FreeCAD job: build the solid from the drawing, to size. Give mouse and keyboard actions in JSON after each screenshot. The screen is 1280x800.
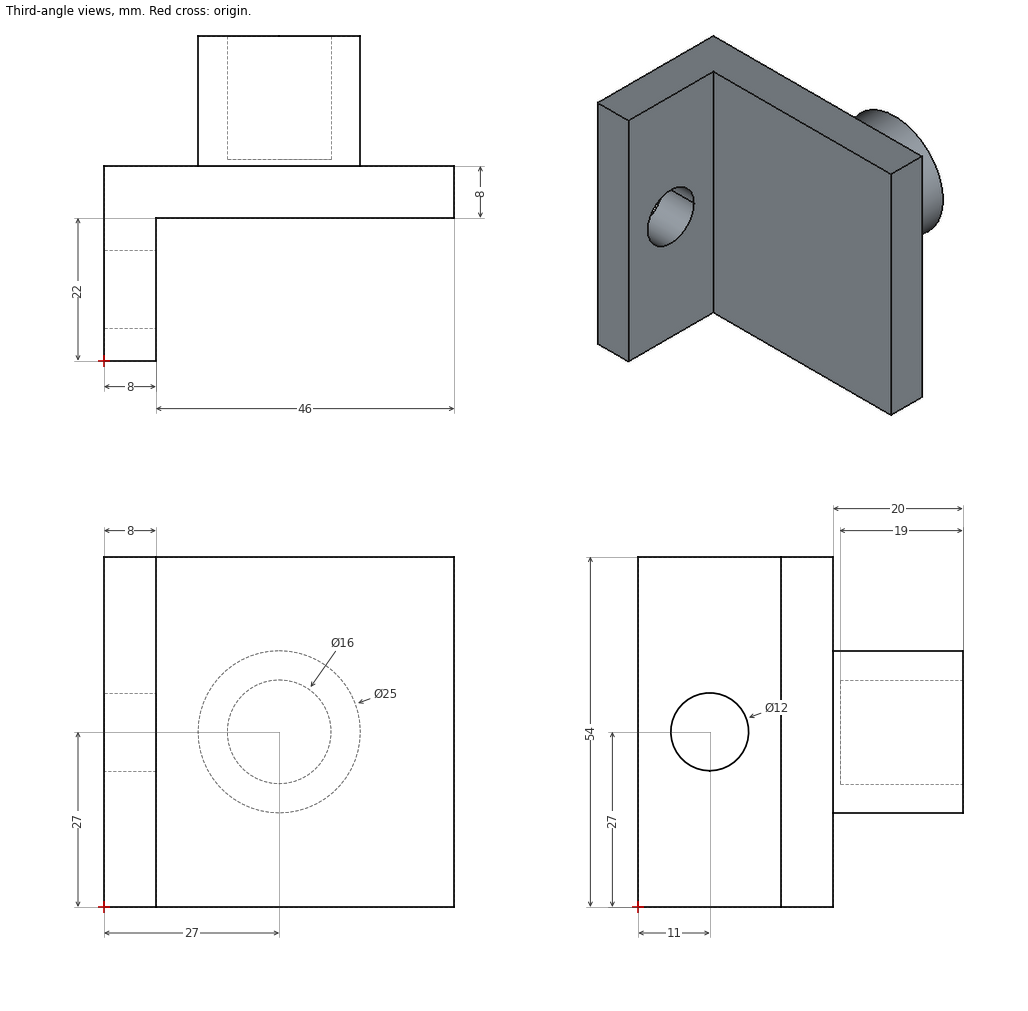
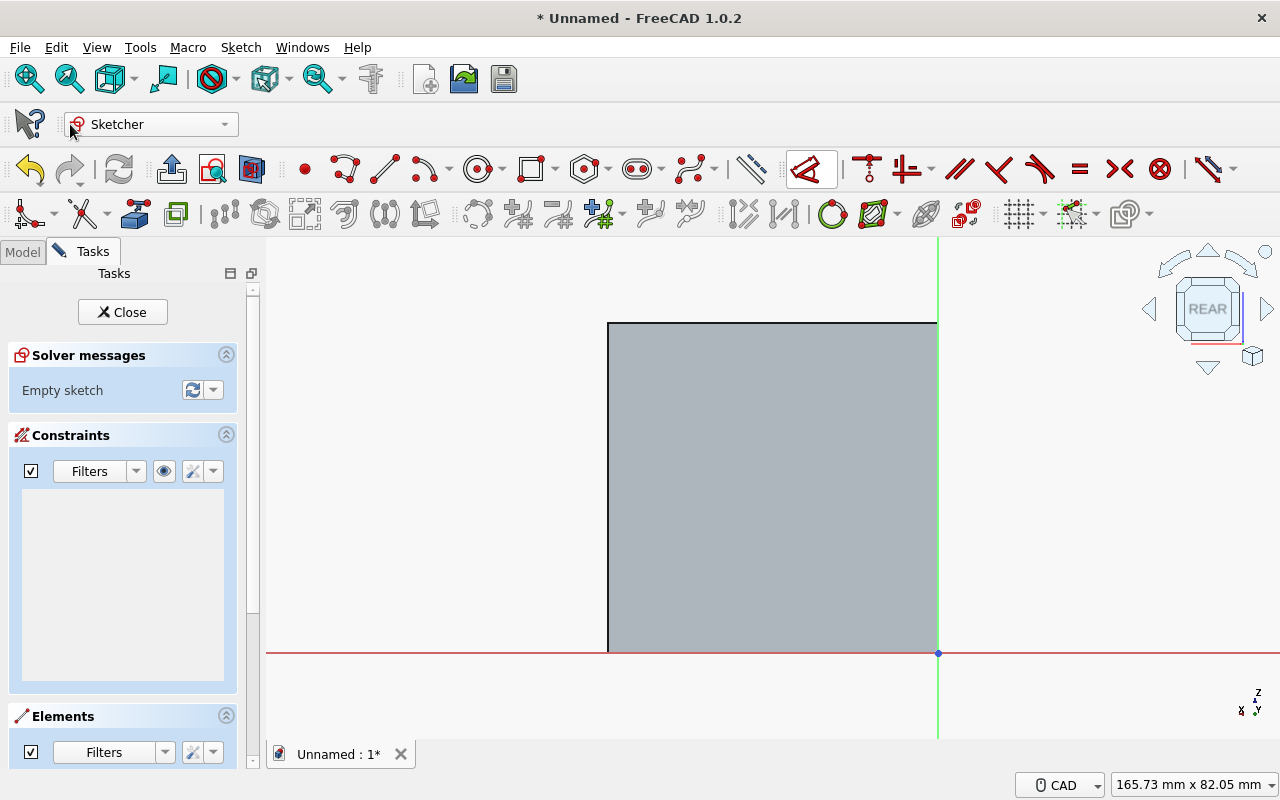
{"action": "key", "text": "g c"}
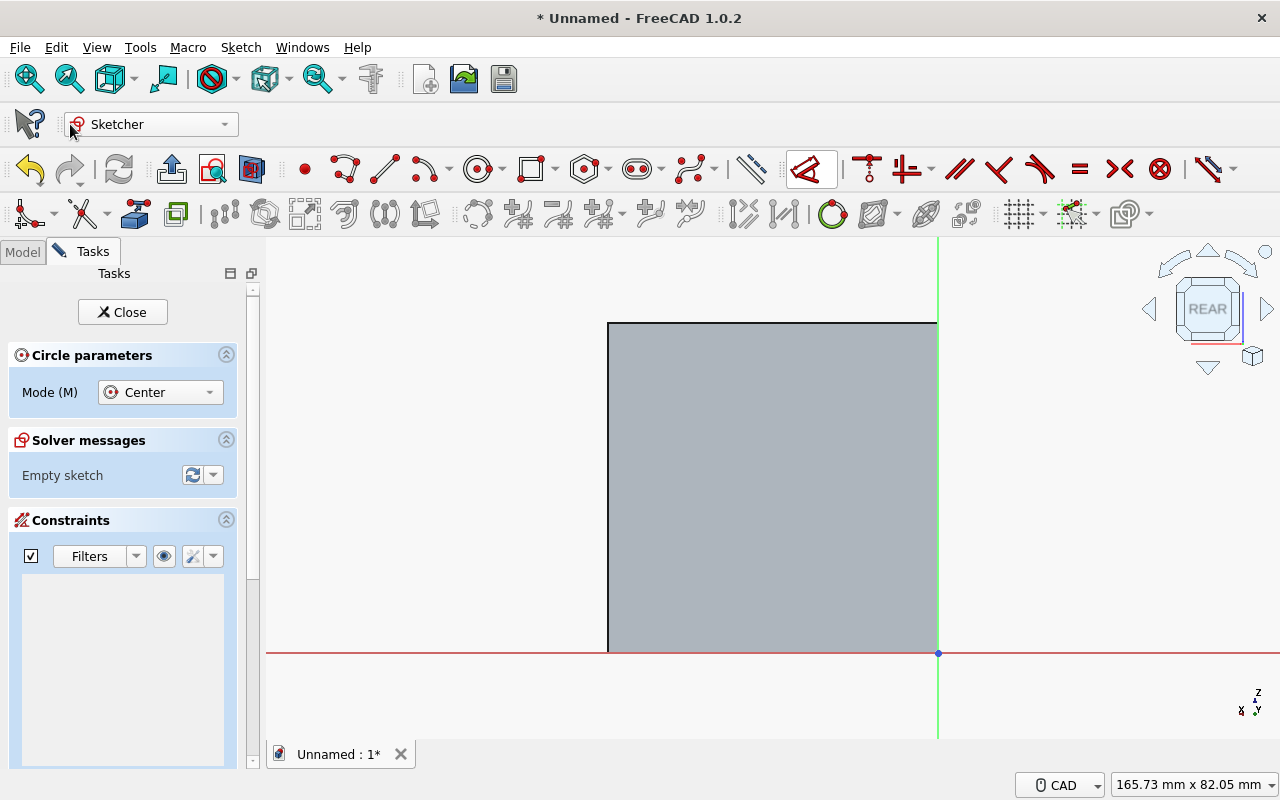
{"action": "left_click", "coordinate": [773, 488]}
{"action": "mouse_move", "coordinate": [827, 434]}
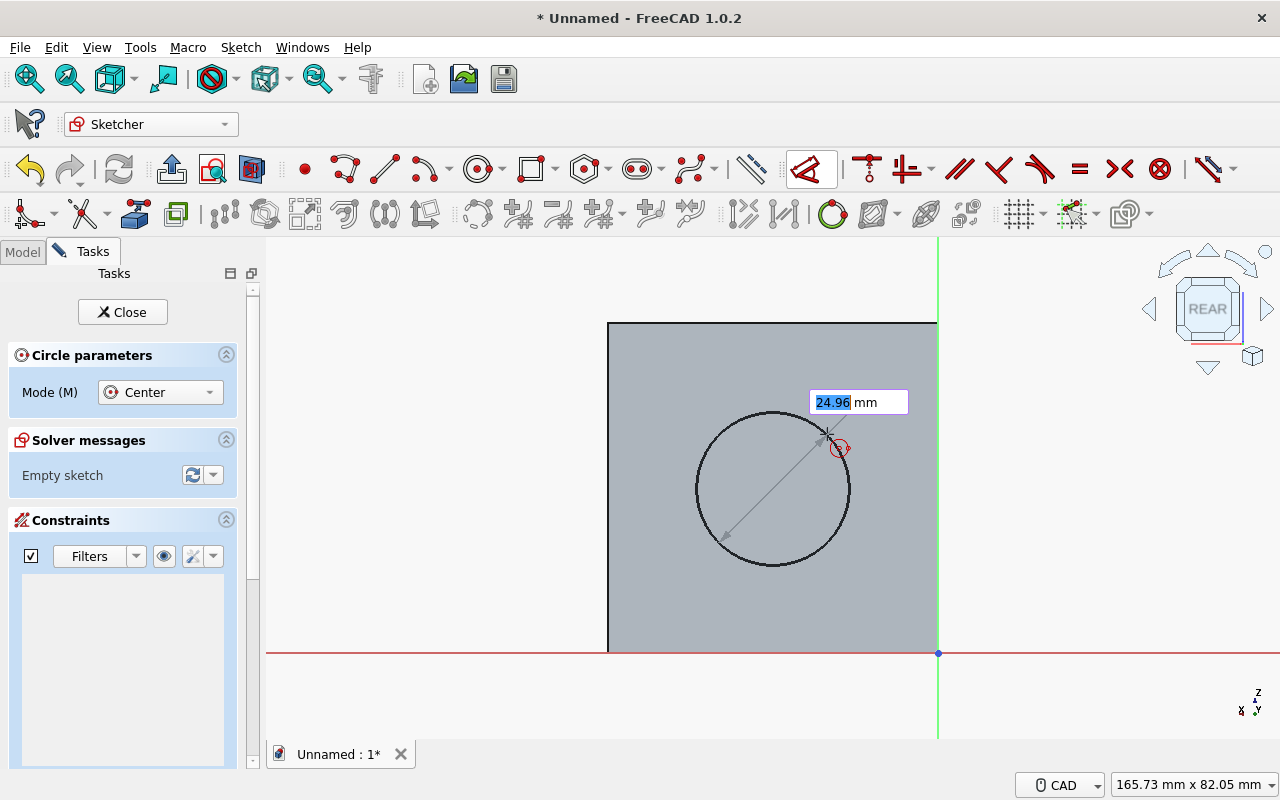
{"action": "type", "text": "25"}
{"action": "key", "text": "Return"}
{"action": "key", "text": "Escape"}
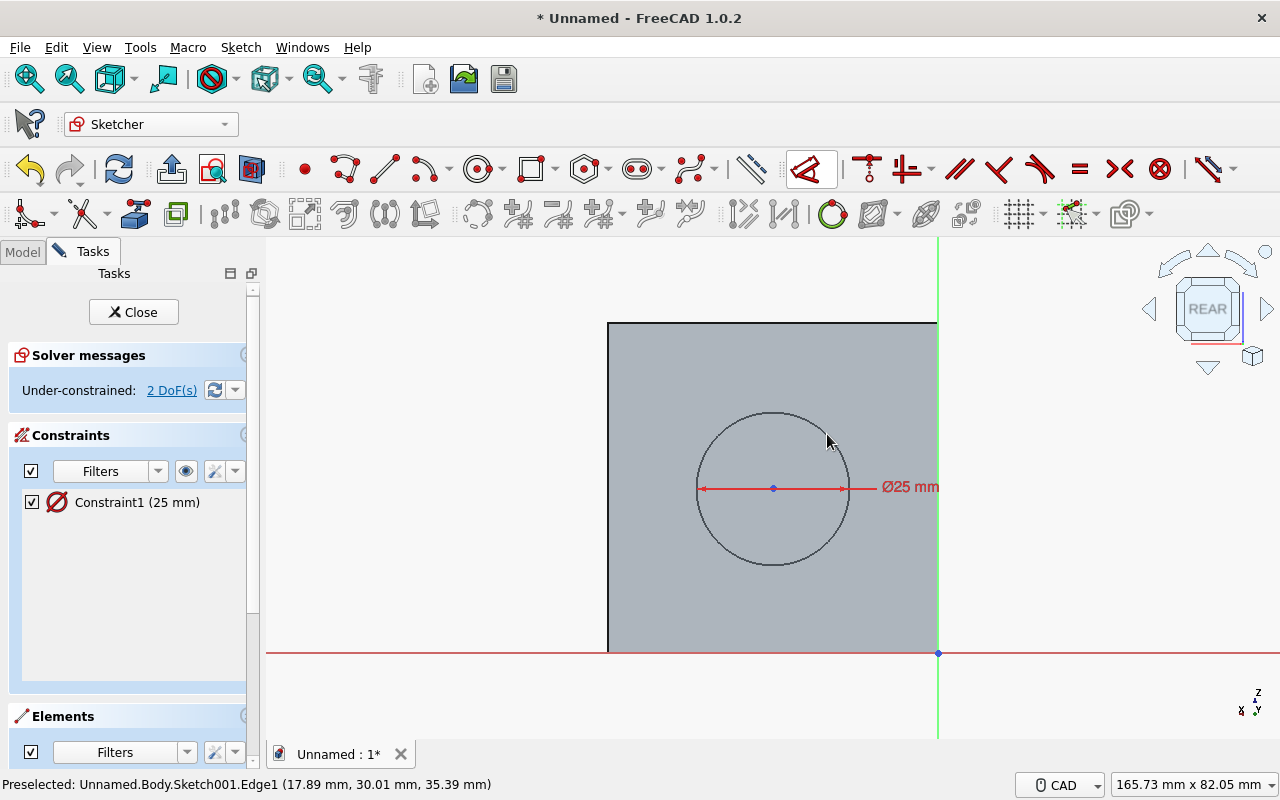
{"action": "left_click", "coordinate": [773, 489]}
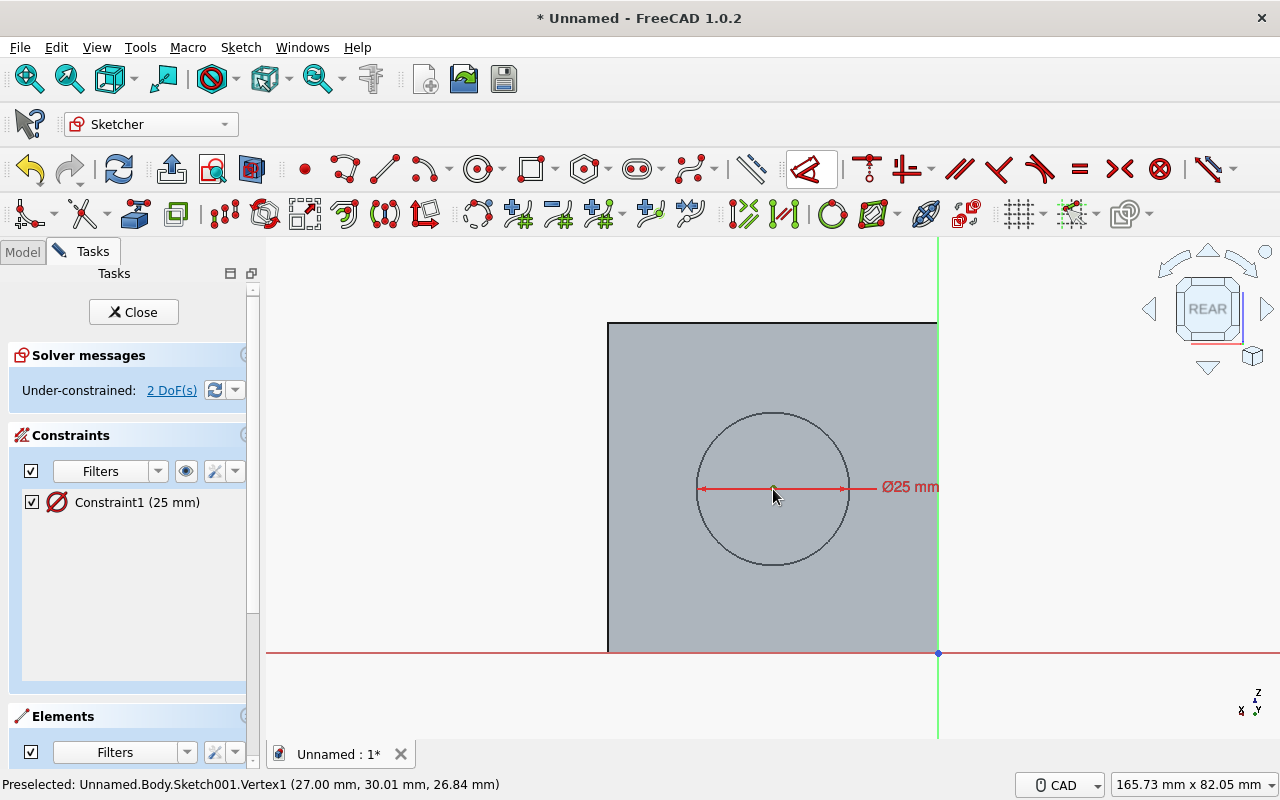
{"action": "key", "text": "l"}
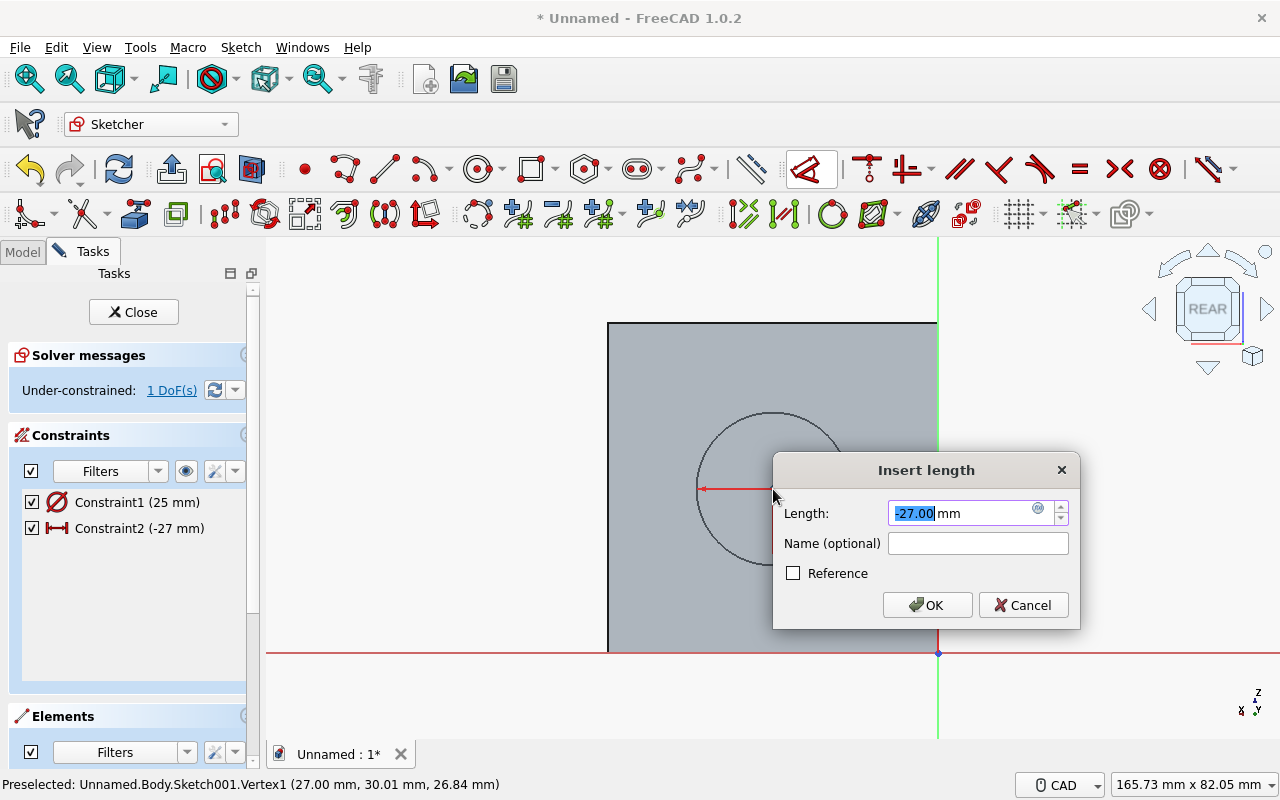
{"action": "type", "text": "-27"}
{"action": "key", "text": "Return"}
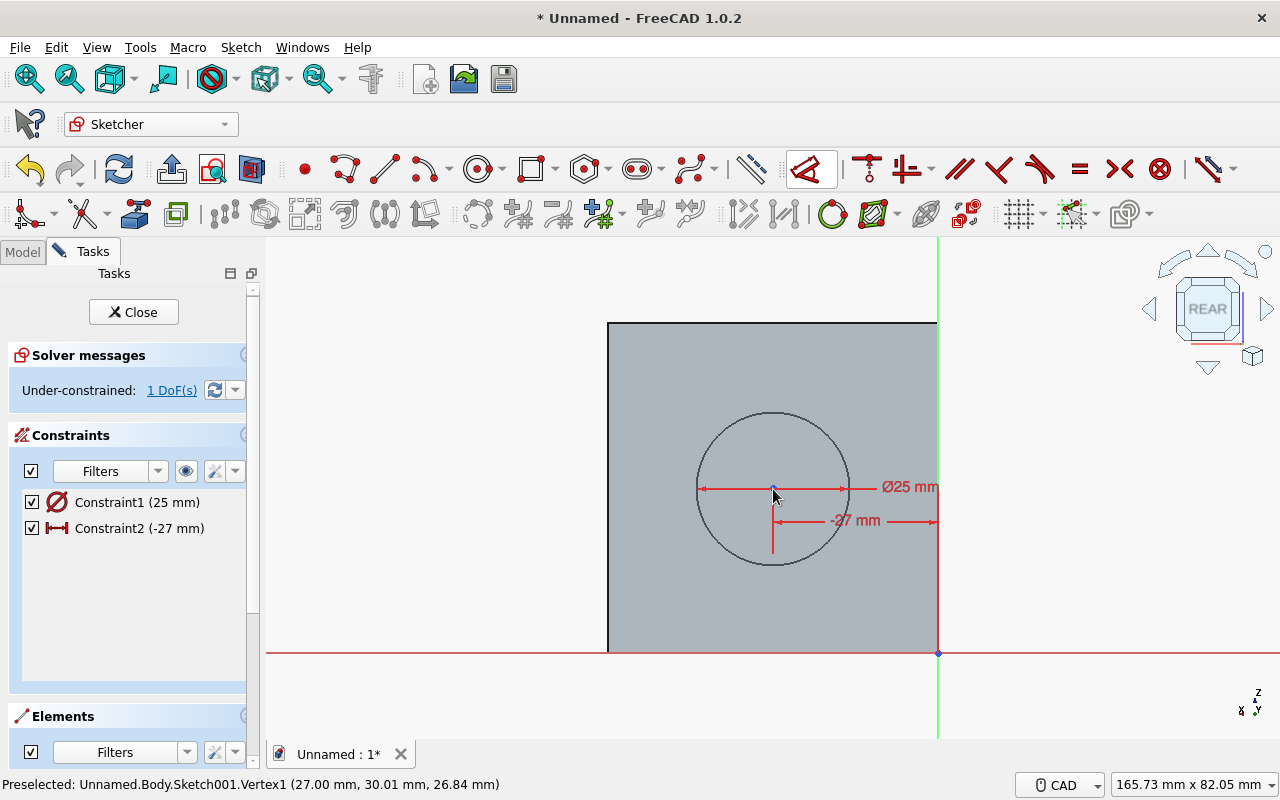
{"action": "left_click", "coordinate": [773, 489]}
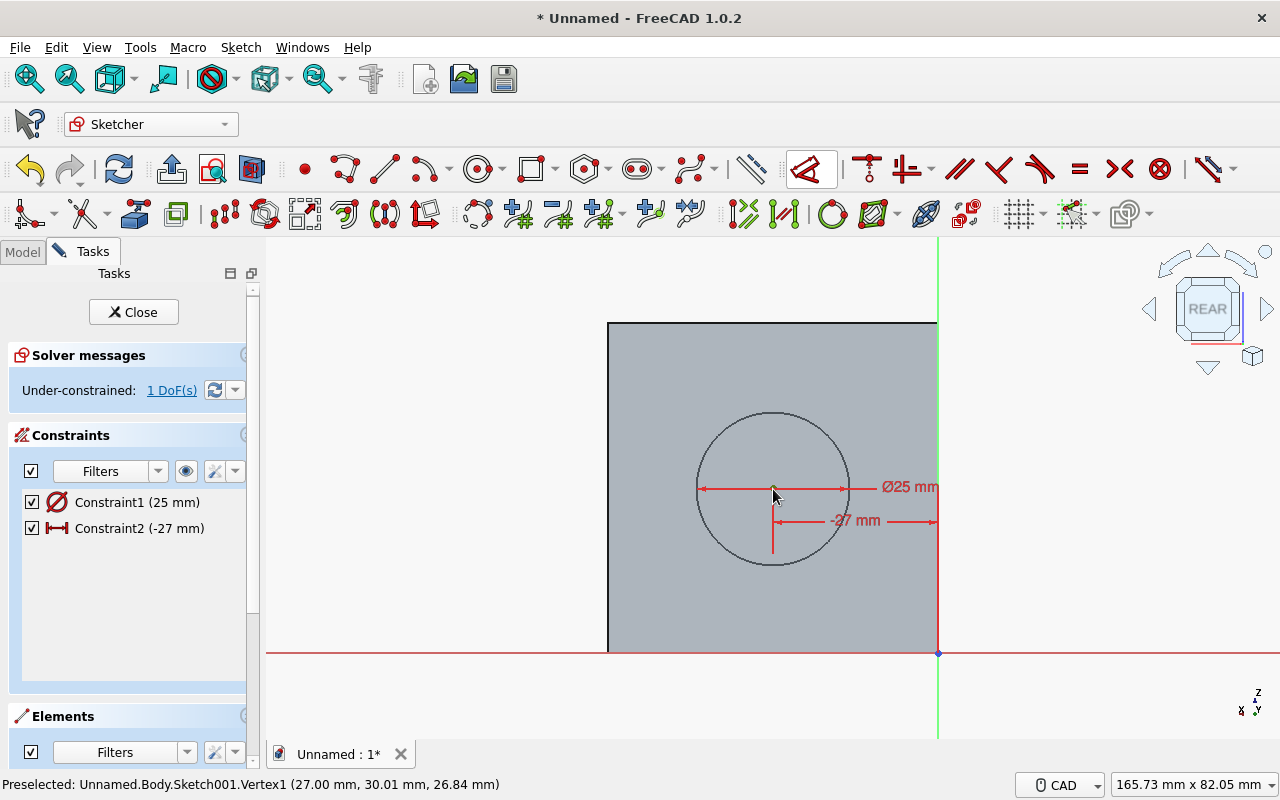
{"action": "key", "text": "i"}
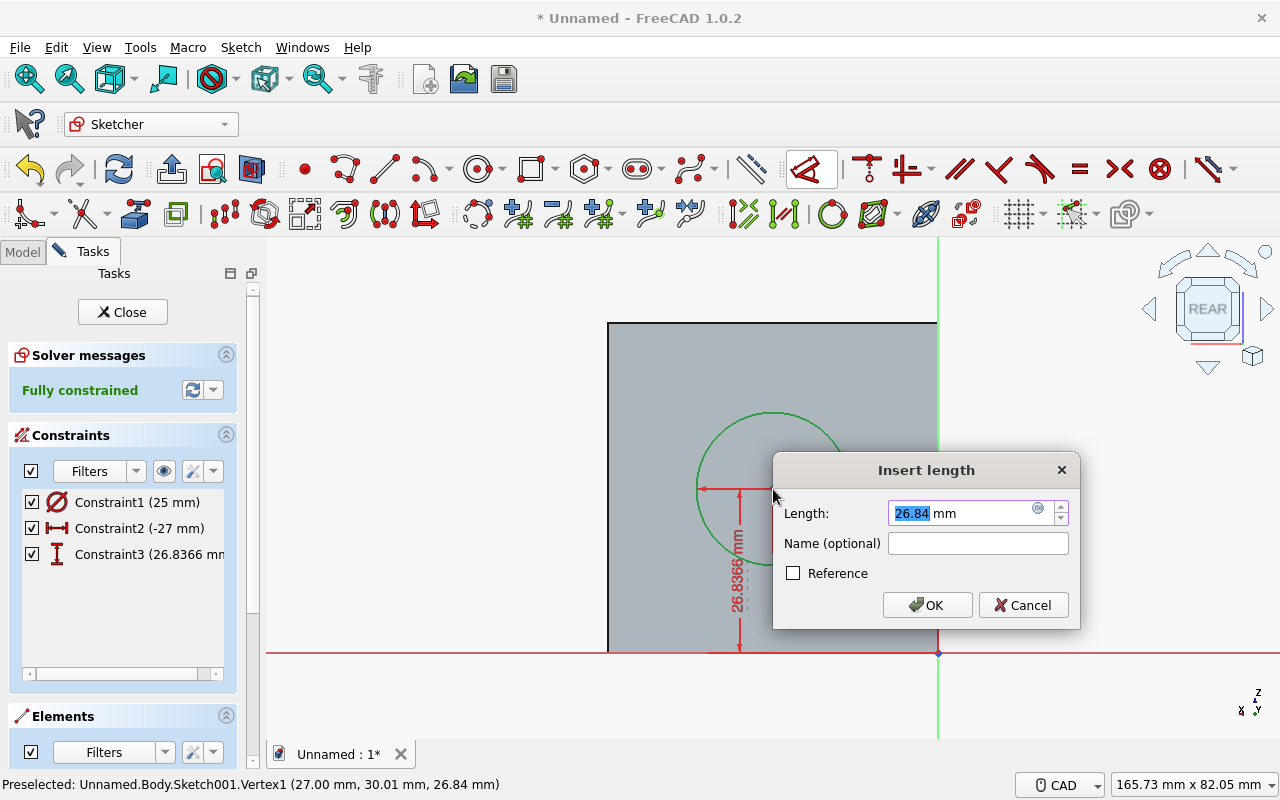
{"action": "type", "text": "27"}
{"action": "key", "text": "Return"}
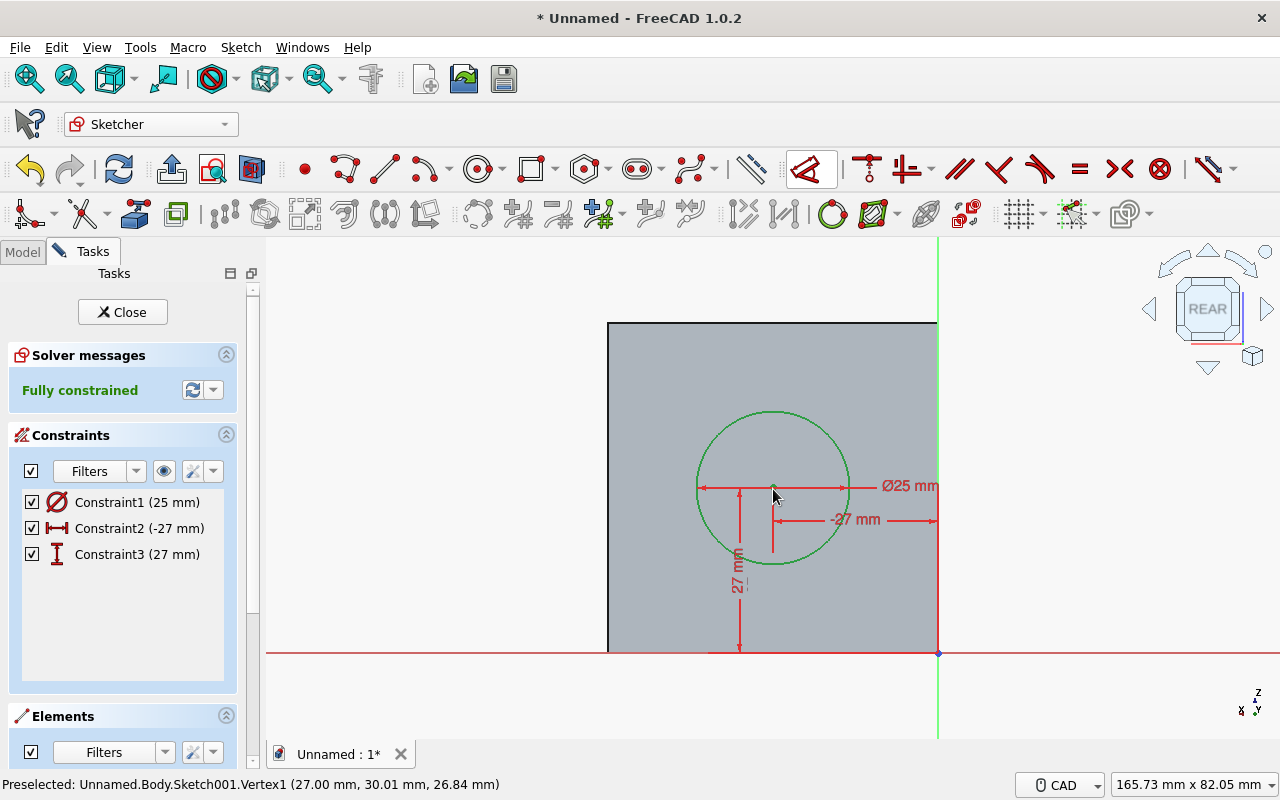
{"action": "left_click", "coordinate": [123, 312]}